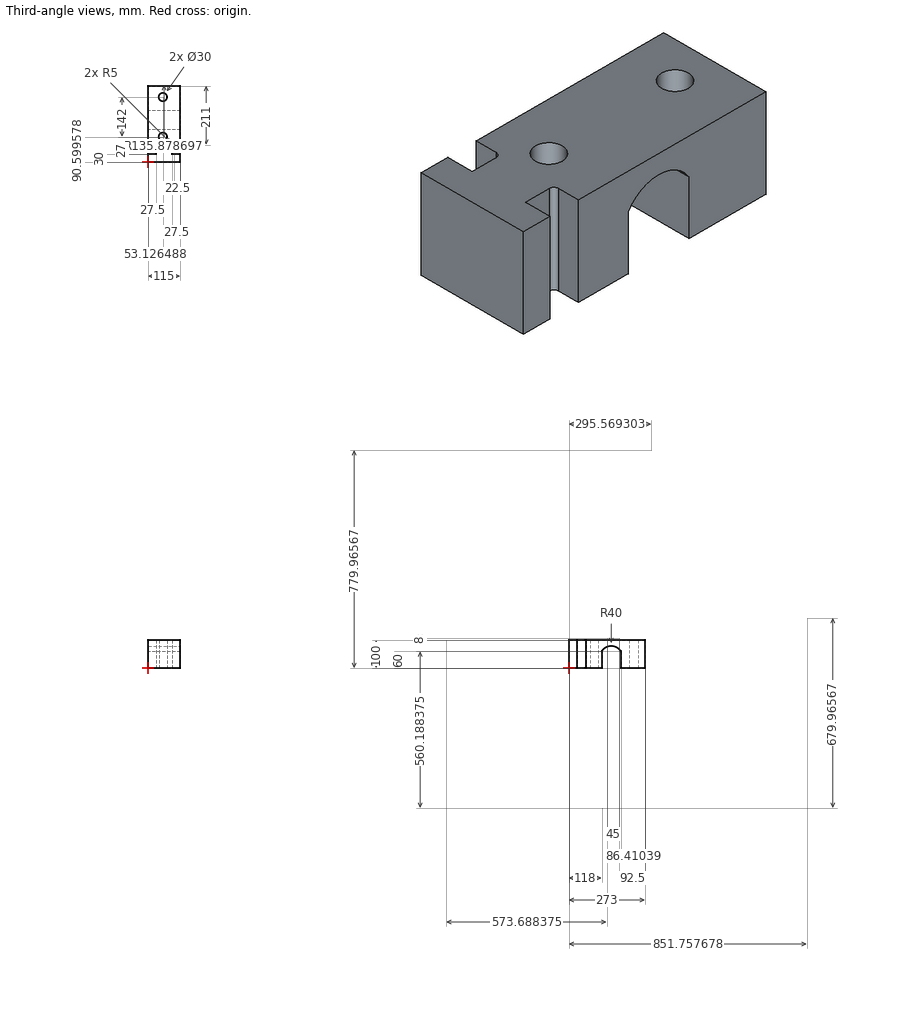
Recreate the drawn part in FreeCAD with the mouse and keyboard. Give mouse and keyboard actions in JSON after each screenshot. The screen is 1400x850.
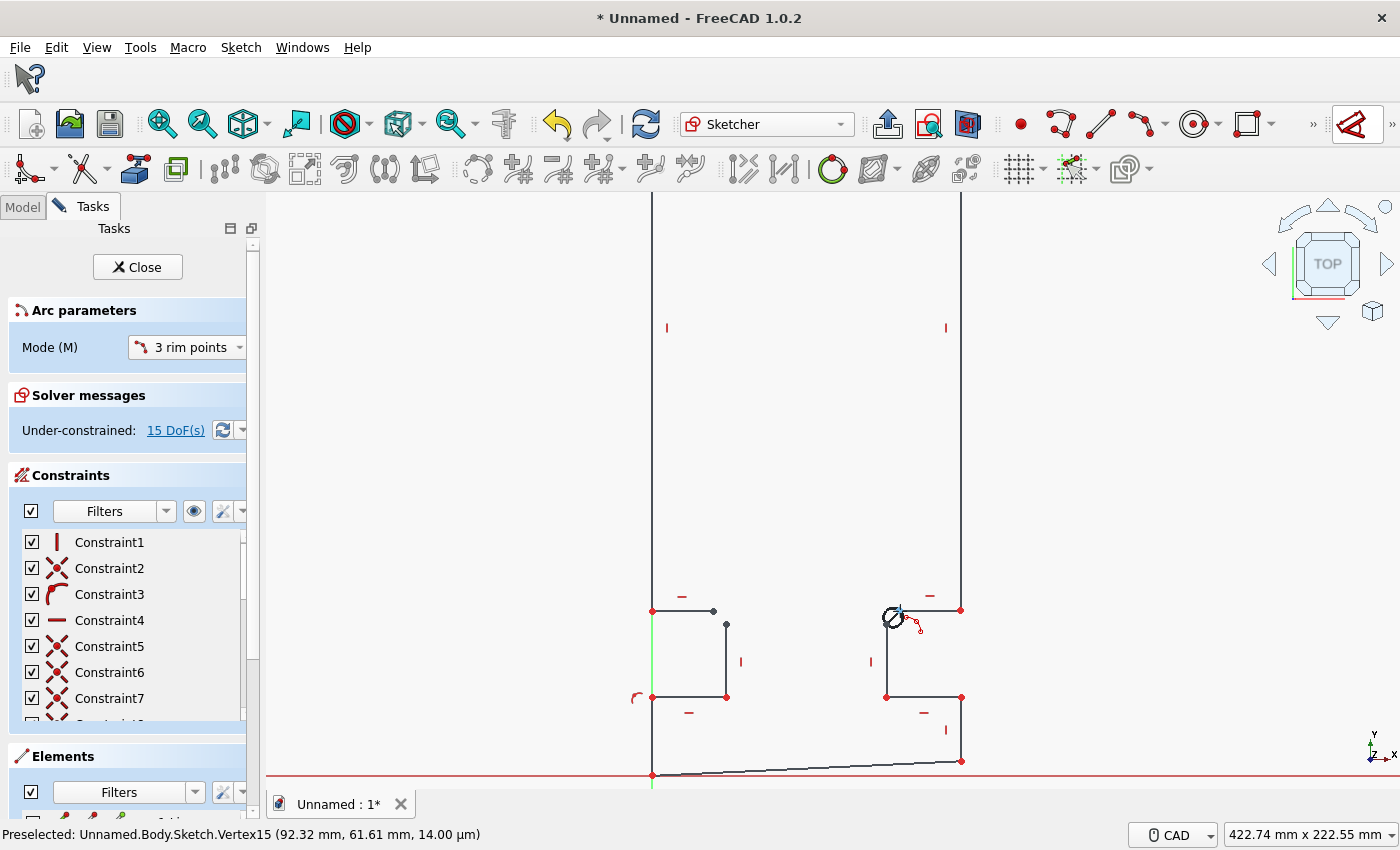
{"action": "scroll", "coordinate": [891, 613], "scroll_direction": "up", "scroll_amount": 7}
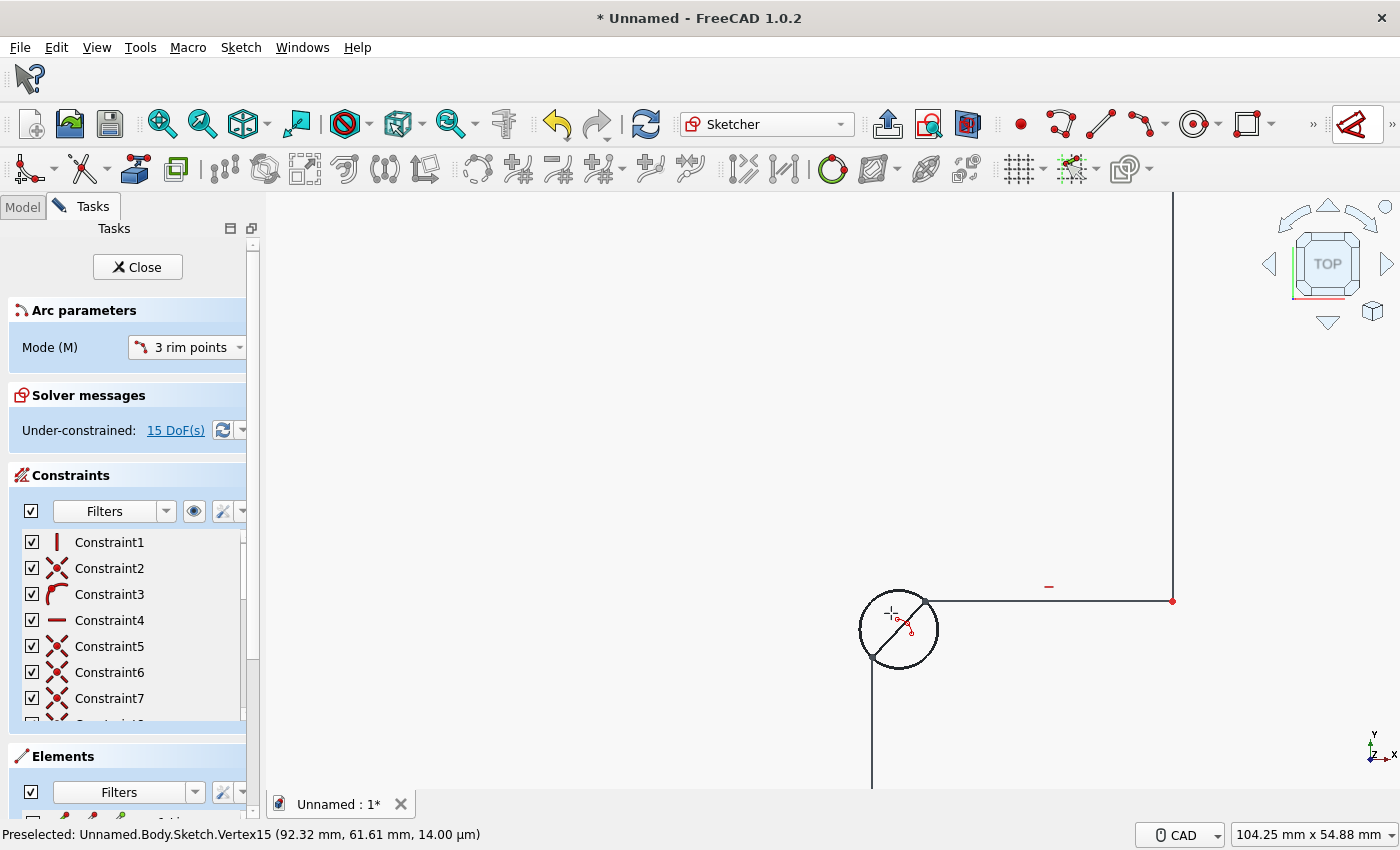
{"action": "left_click", "coordinate": [889, 613]}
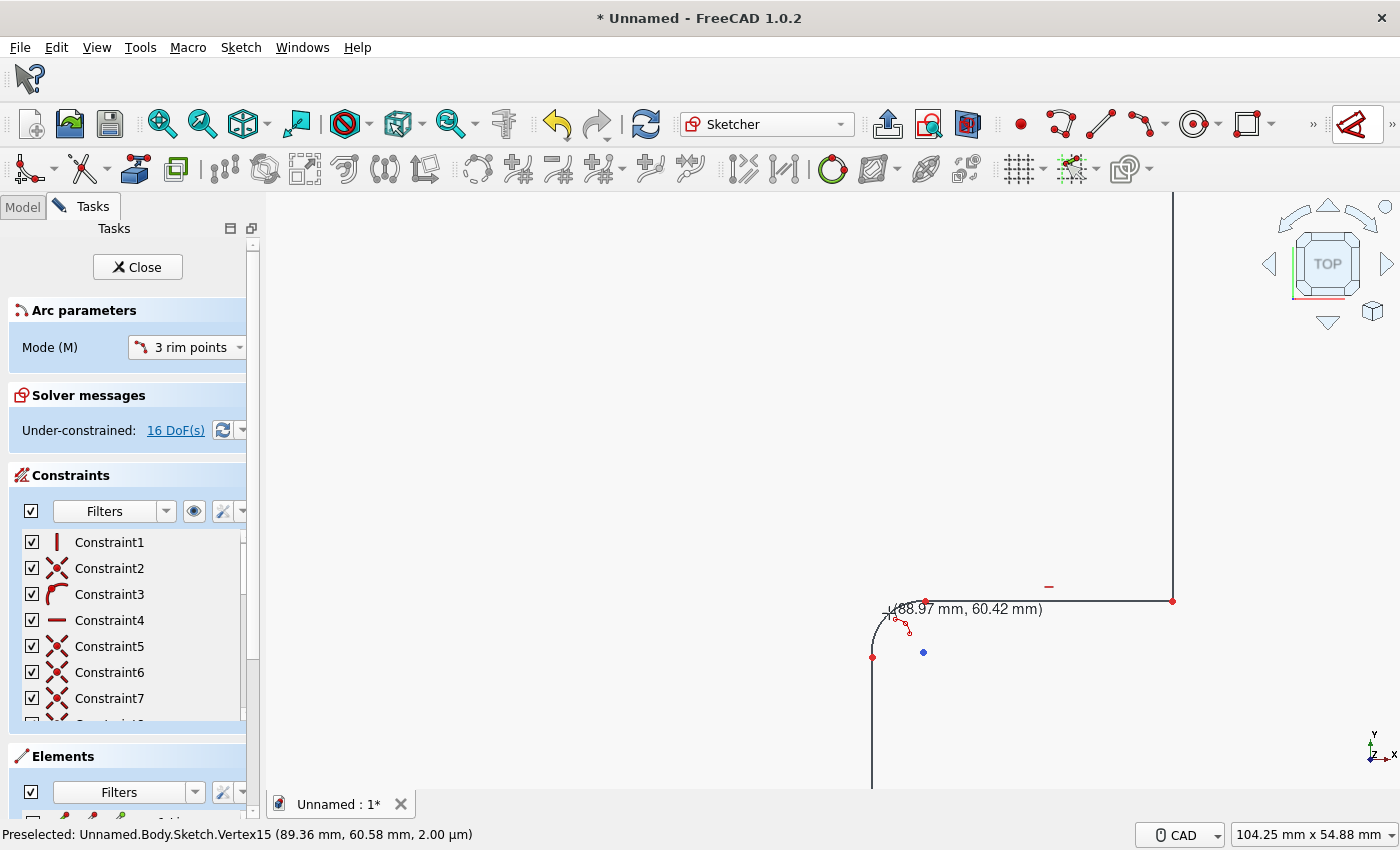
{"action": "scroll", "coordinate": [799, 612], "scroll_direction": "down", "scroll_amount": 10}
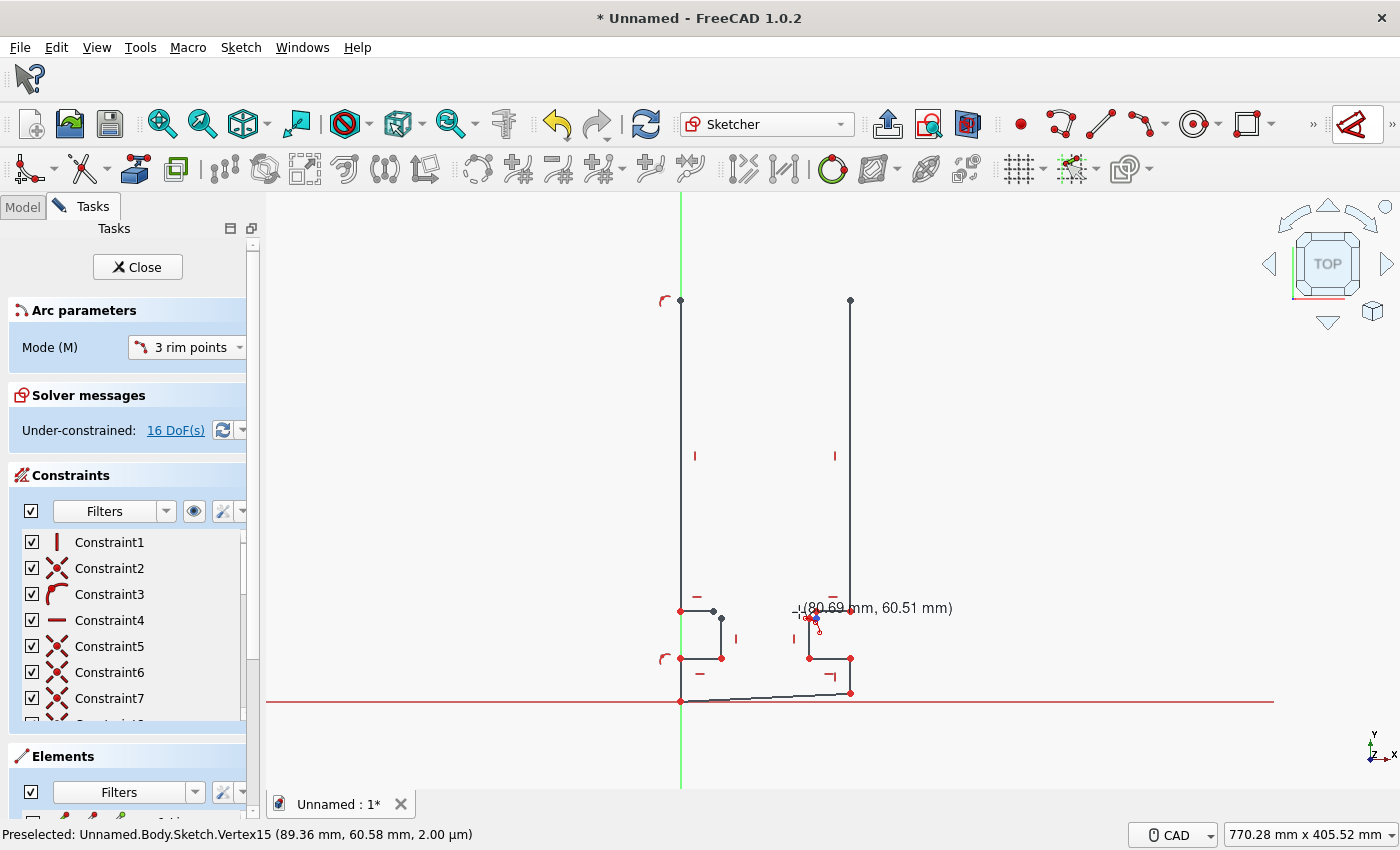
{"action": "left_click", "coordinate": [850, 300]}
{"action": "left_click", "coordinate": [681, 300]}
{"action": "left_click", "coordinate": [765, 281]}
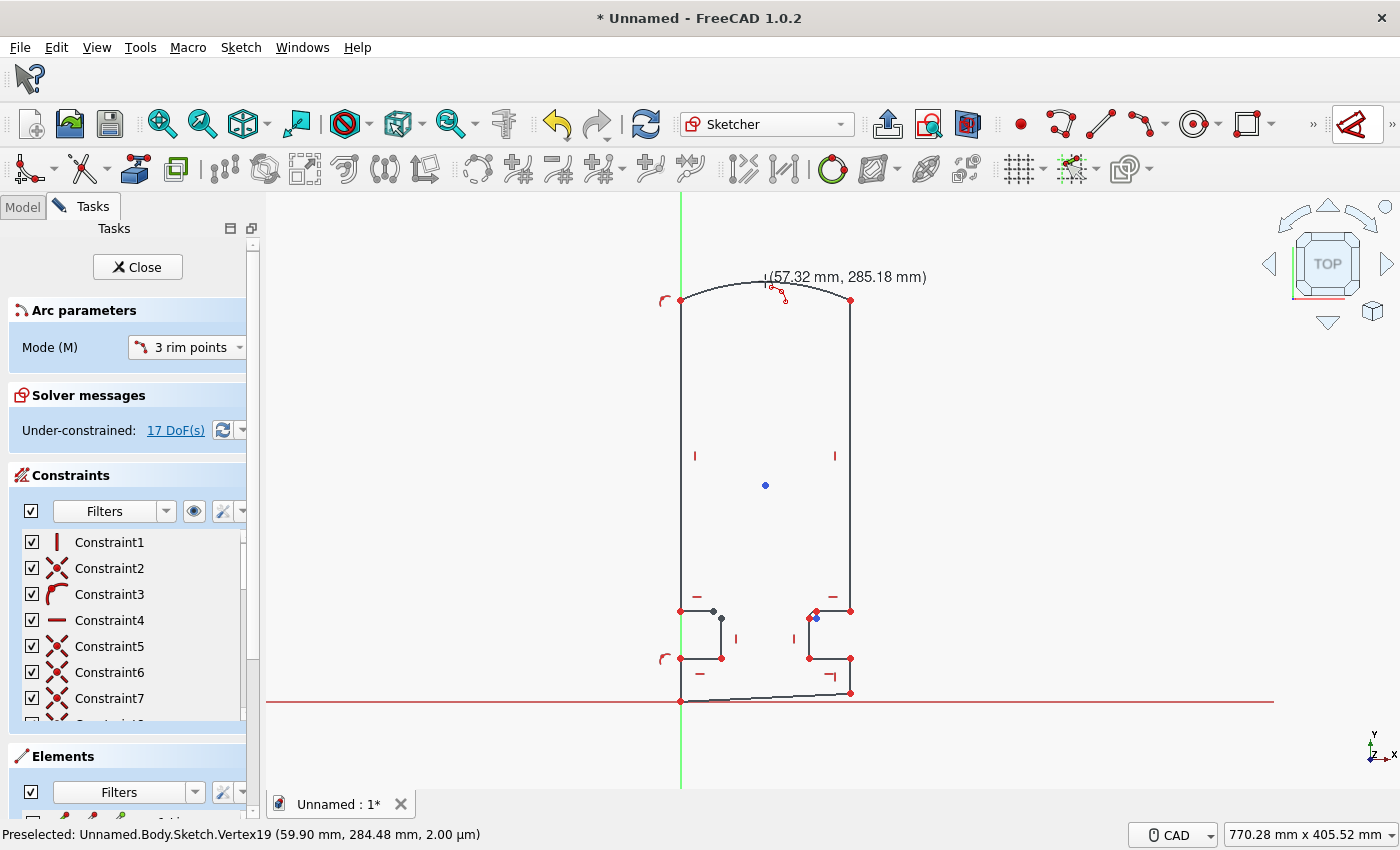
{"action": "scroll", "coordinate": [714, 611], "scroll_direction": "up", "scroll_amount": 3}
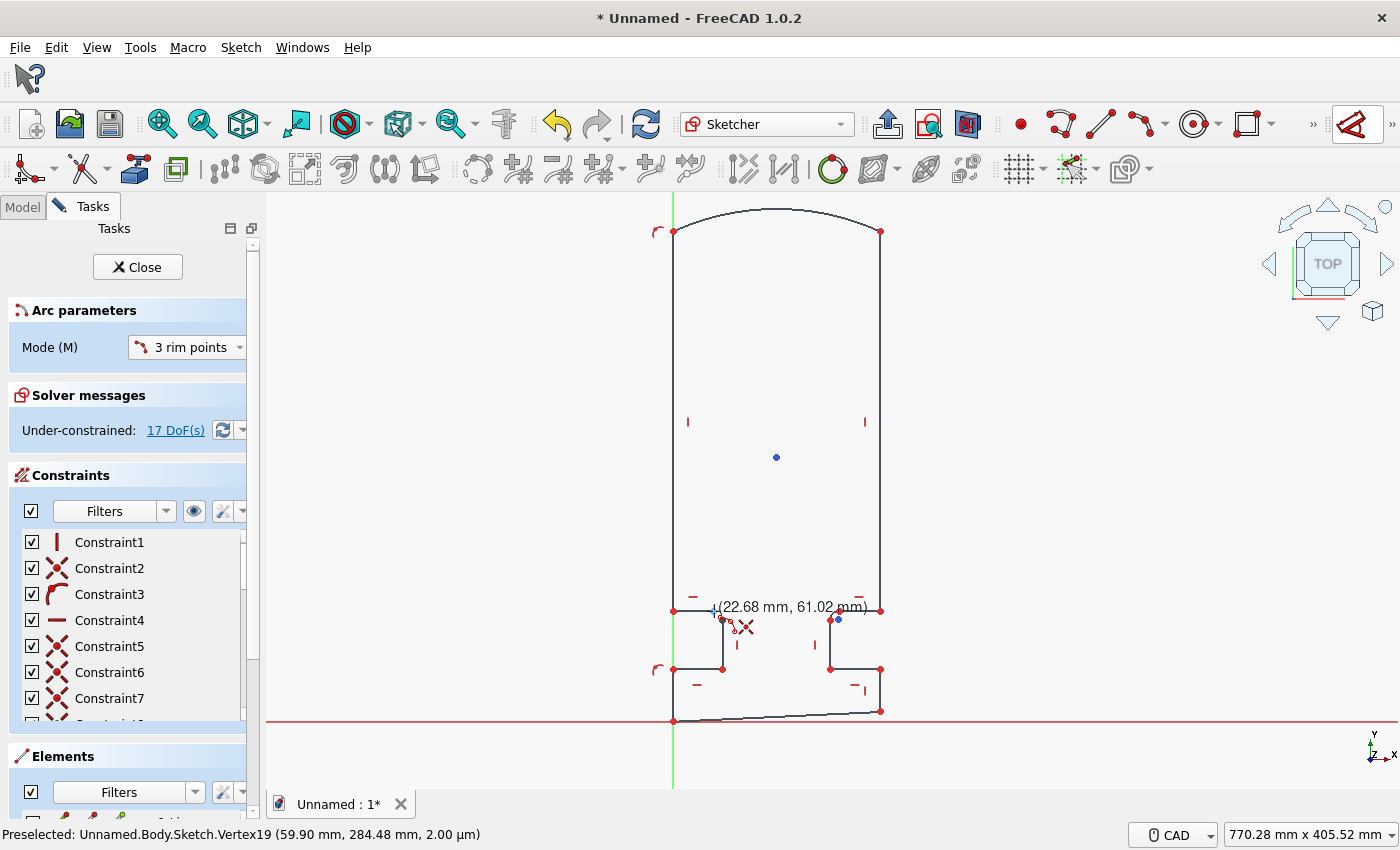
{"action": "left_click", "coordinate": [714, 611]}
{"action": "left_click", "coordinate": [727, 625]}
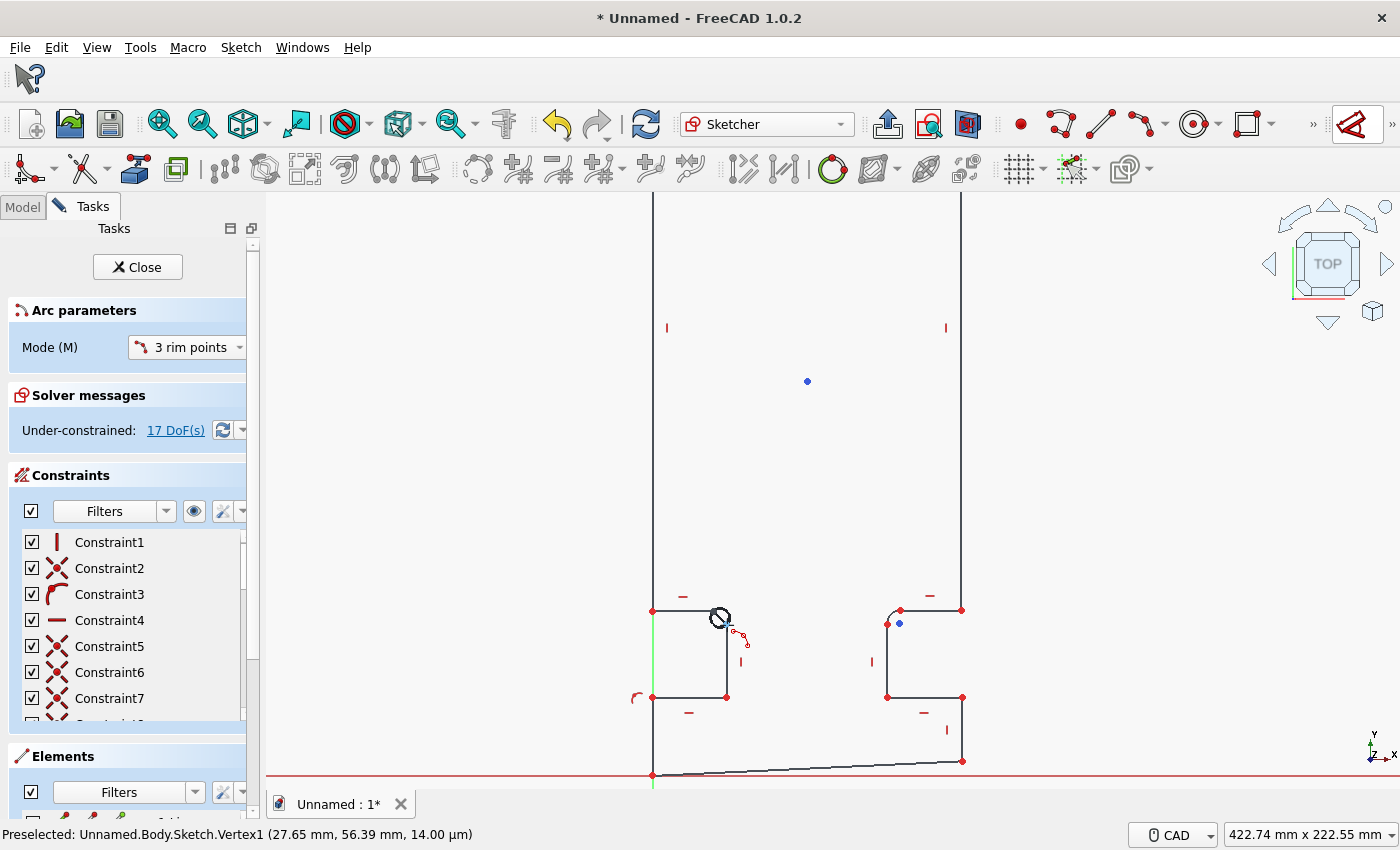
{"action": "scroll", "coordinate": [723, 614], "scroll_direction": "up", "scroll_amount": 7}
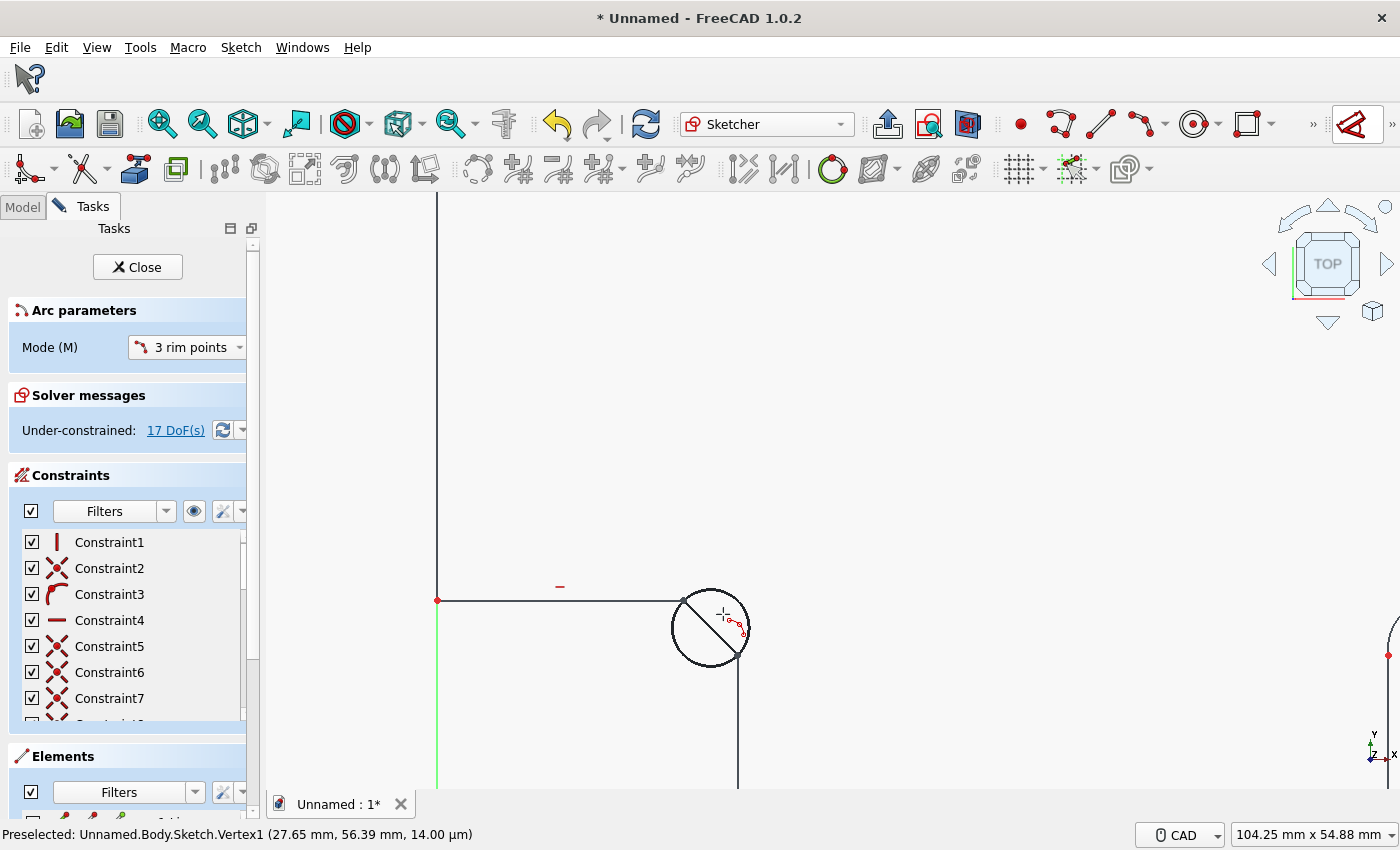
{"action": "left_click", "coordinate": [720, 610]}
{"action": "key", "text": "Escape"}